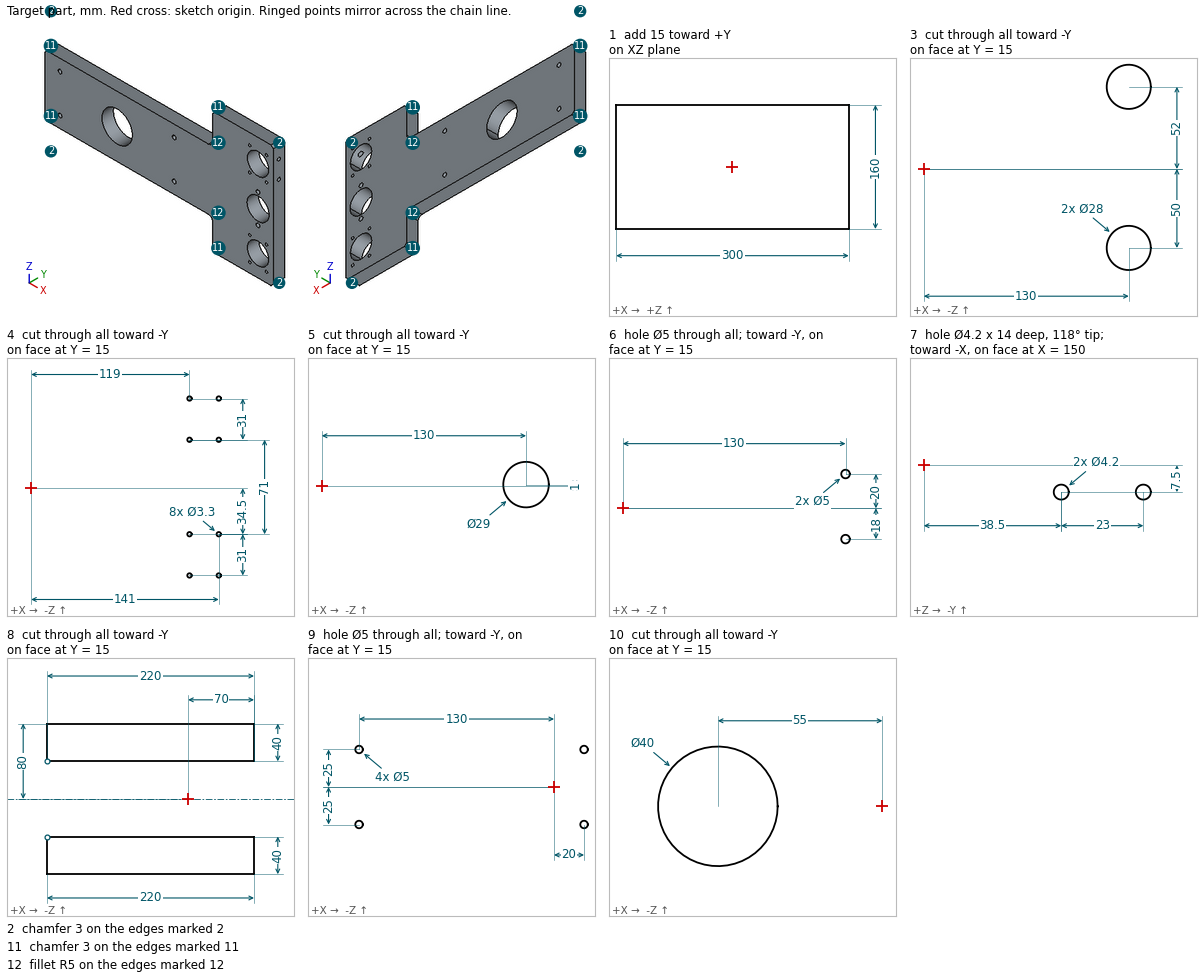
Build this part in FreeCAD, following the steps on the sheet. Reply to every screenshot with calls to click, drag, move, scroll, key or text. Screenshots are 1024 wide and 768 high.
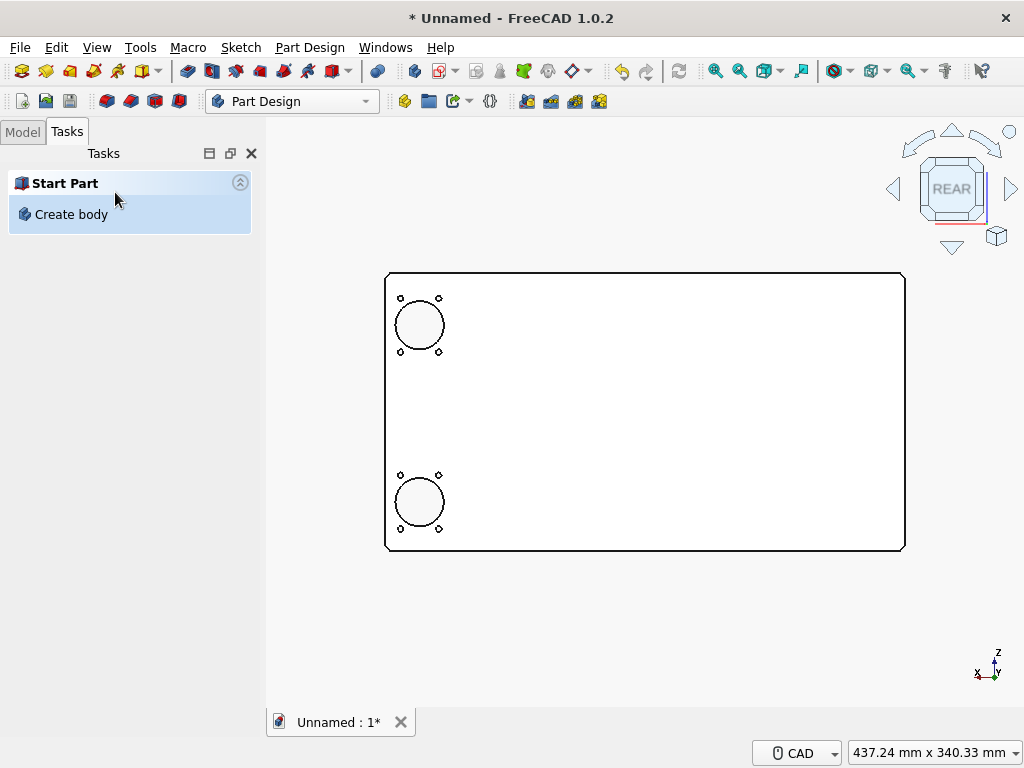
click(571, 411)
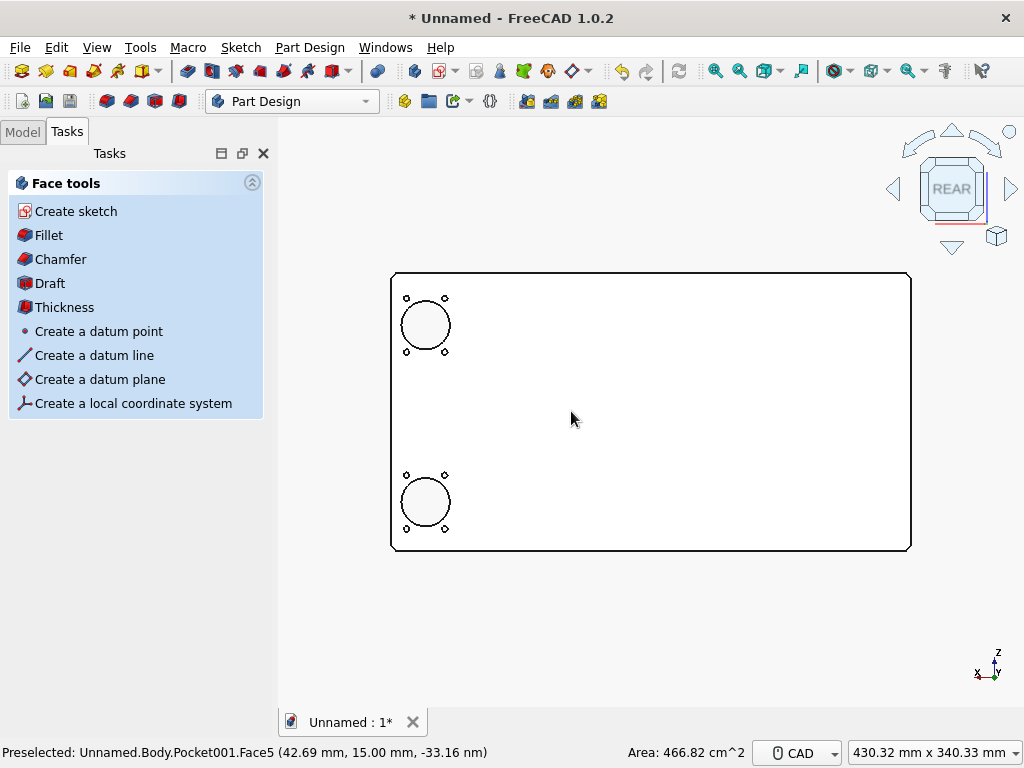
click(440, 72)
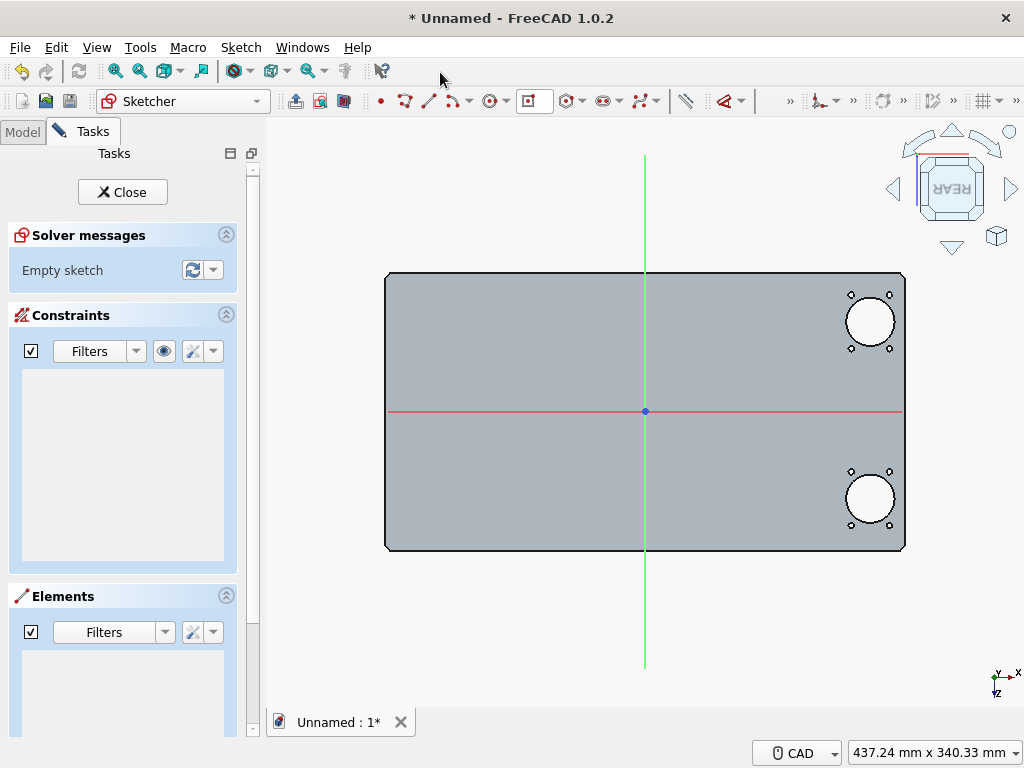
scroll(576, 412, down, 5)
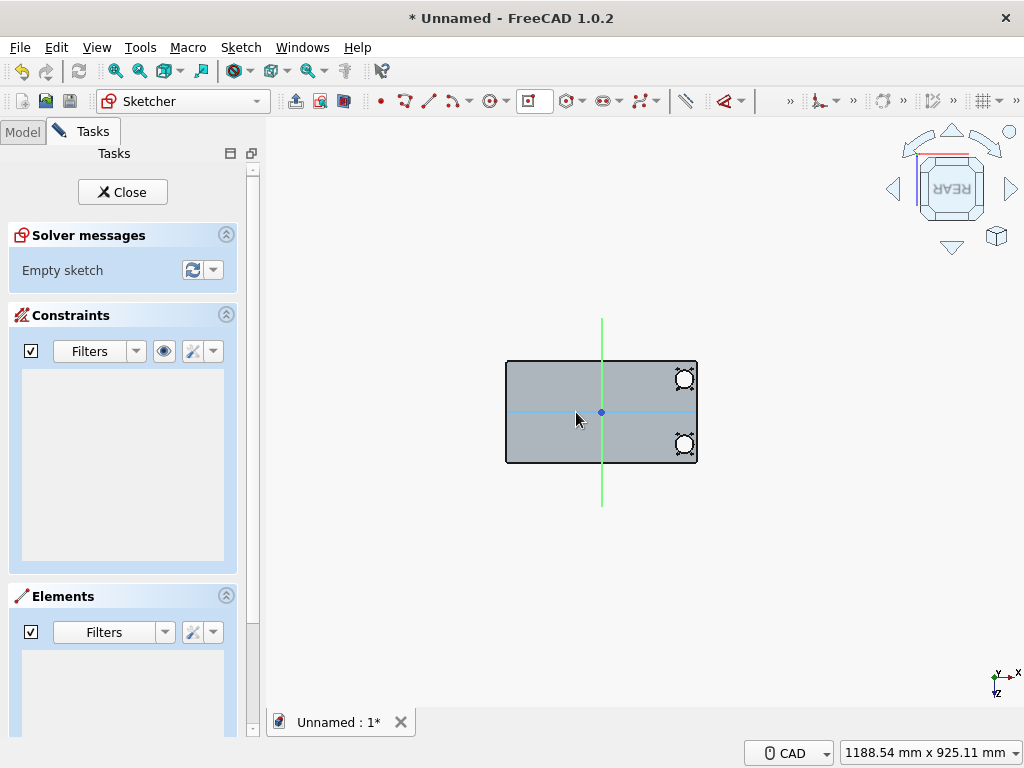
scroll(690, 412, up, 15)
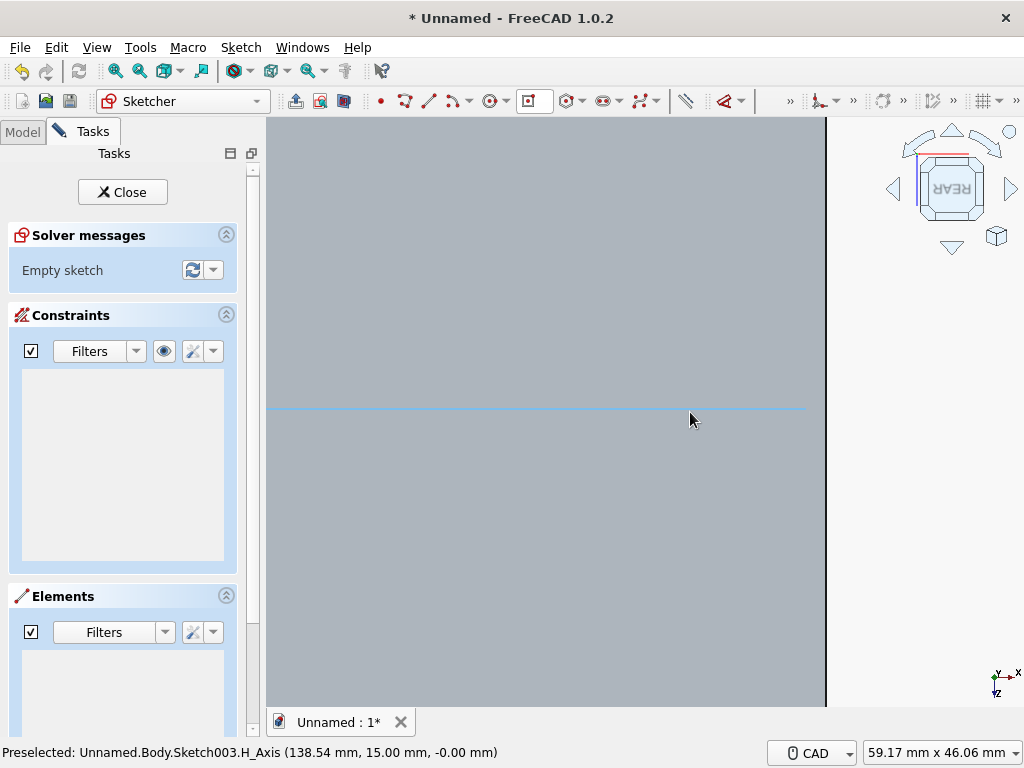
click(490, 102)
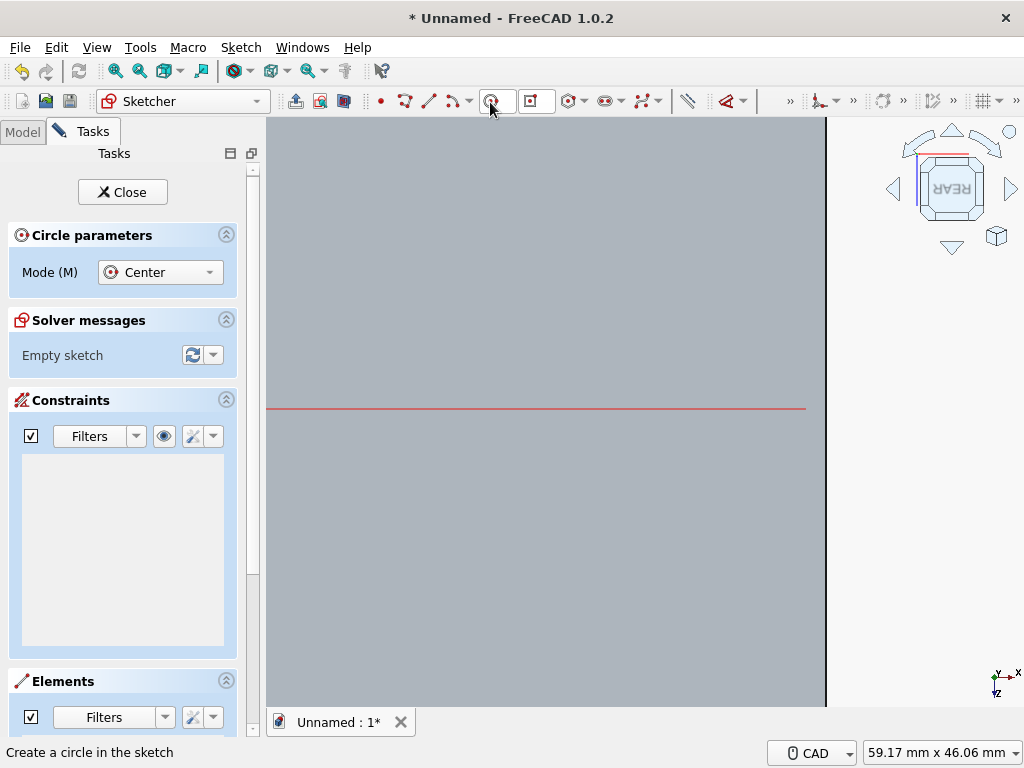
scroll(570, 396, up, 2)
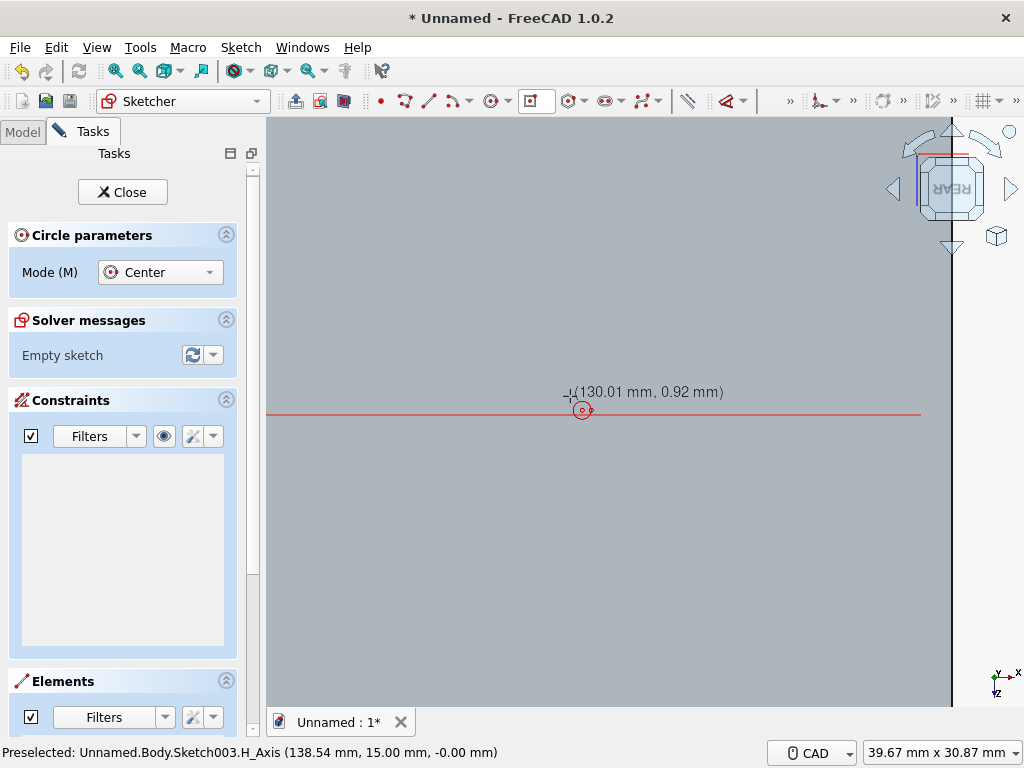
click(570, 396)
move(766, 200)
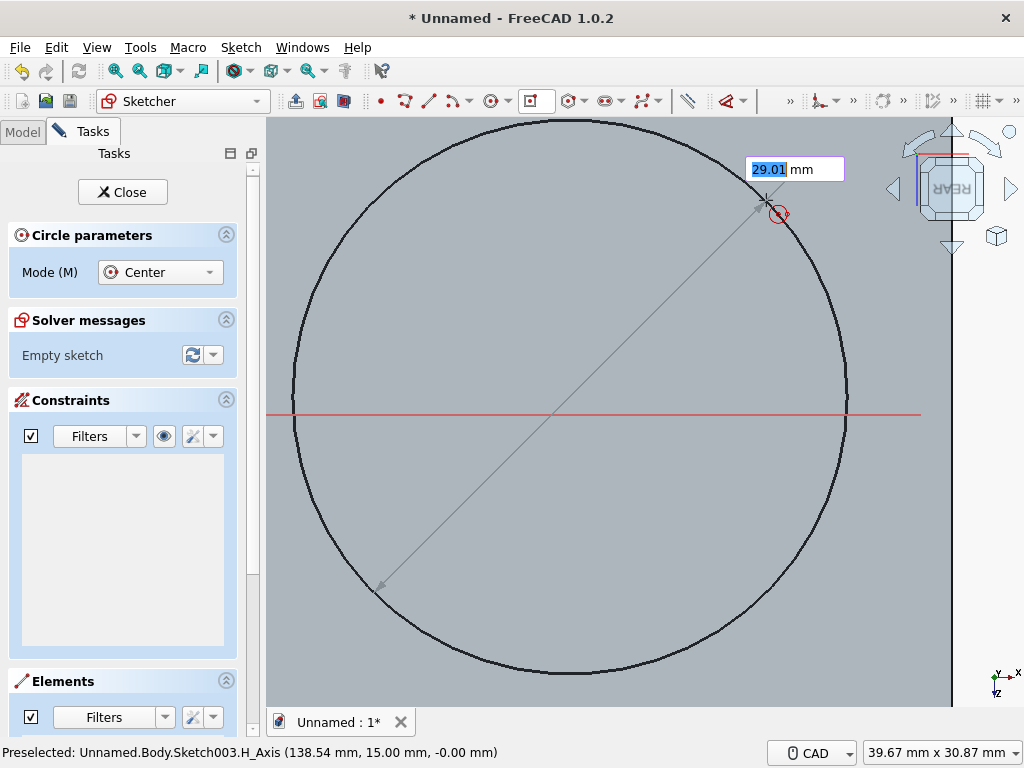
text(29)
key(Return)
key(Escape)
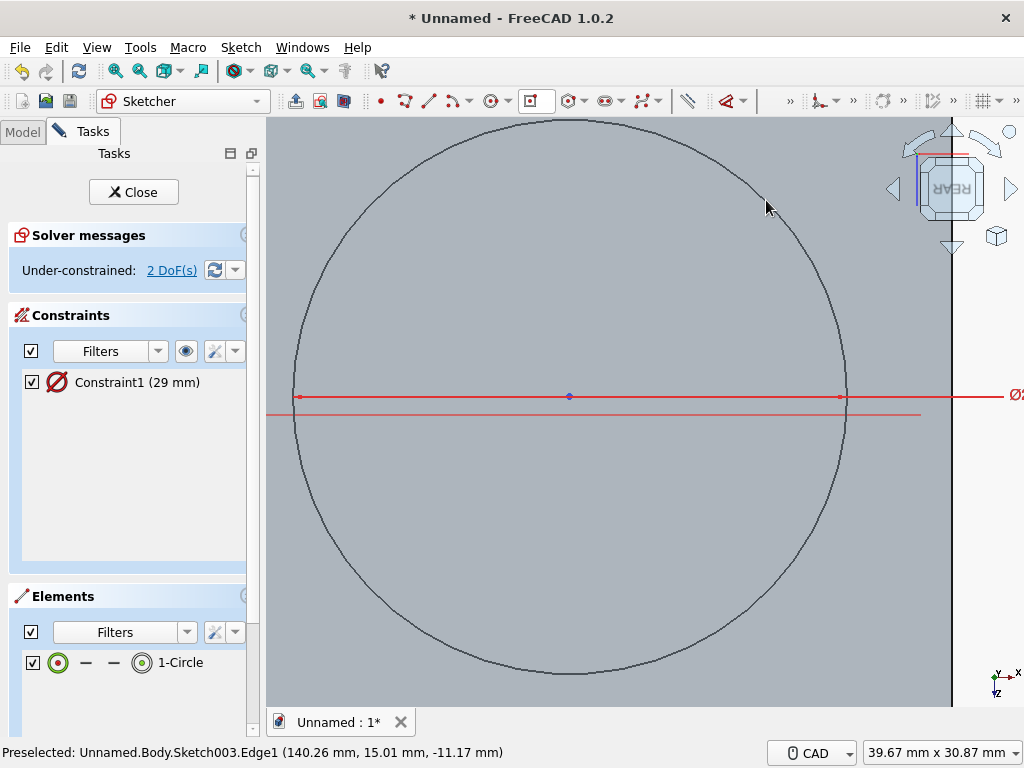
click(726, 102)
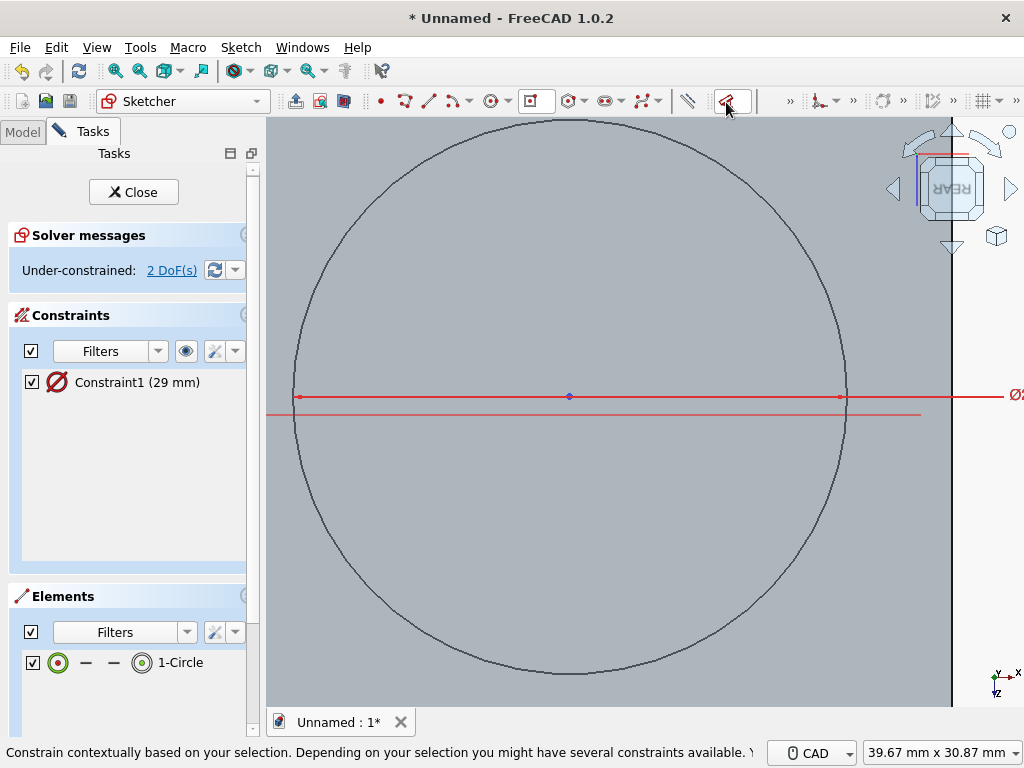
scroll(570, 397, up, 4)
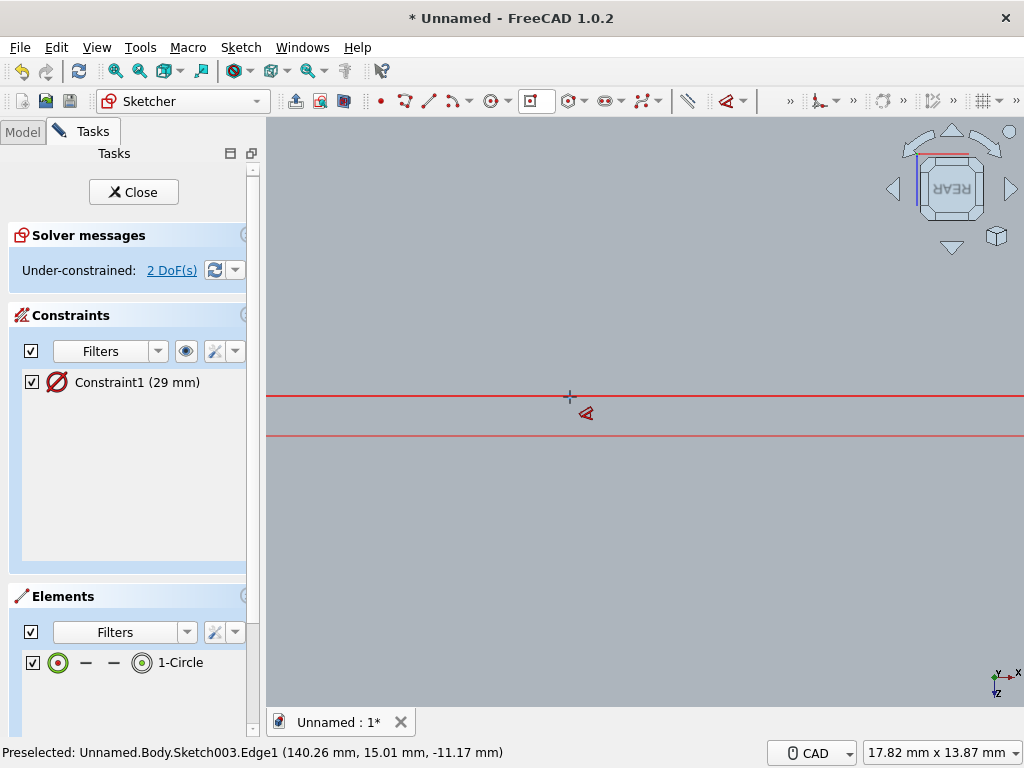
click(570, 396)
click(604, 416)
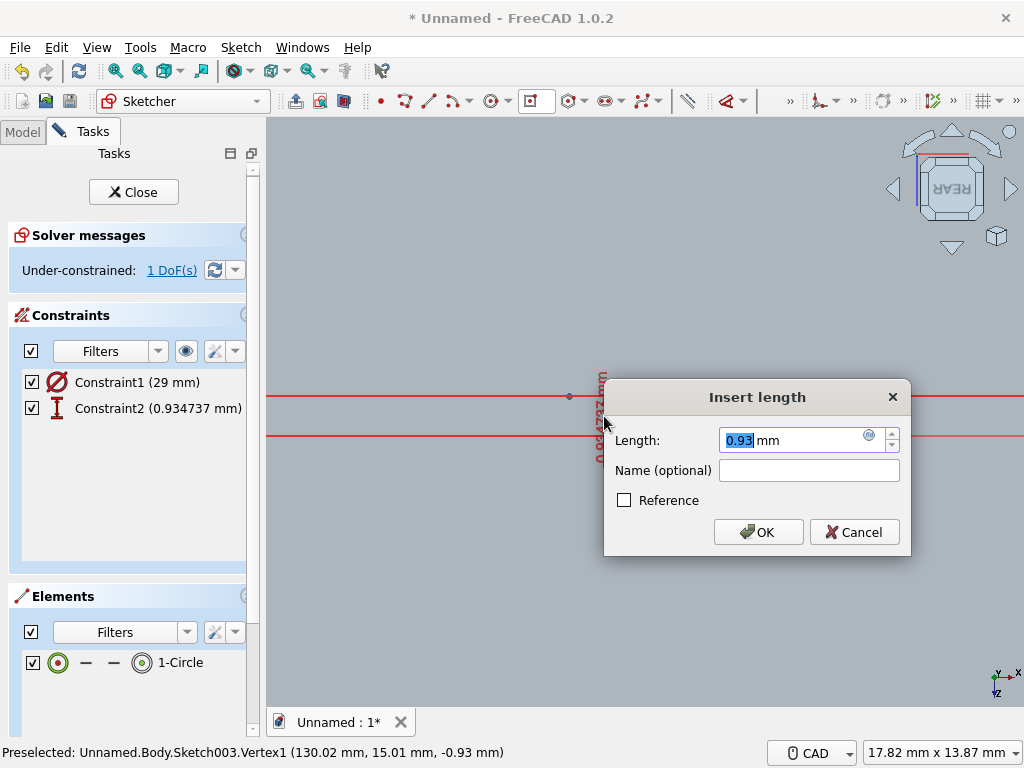
text(1)
key(Return)